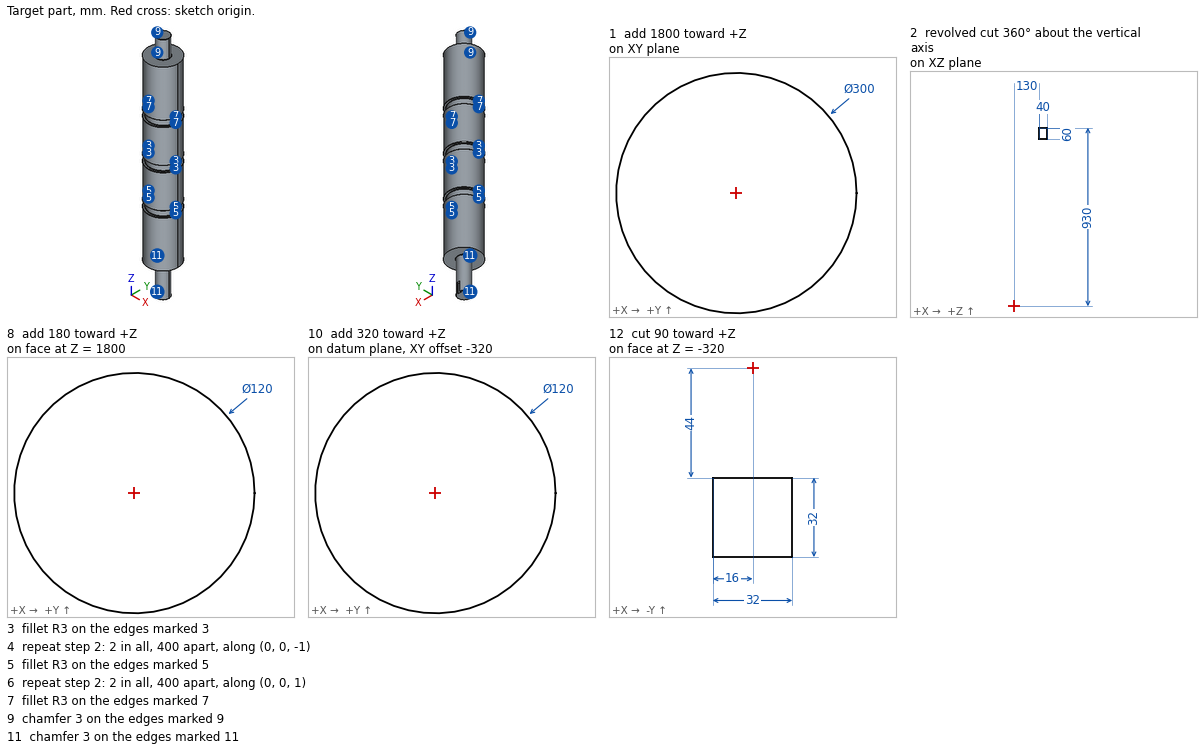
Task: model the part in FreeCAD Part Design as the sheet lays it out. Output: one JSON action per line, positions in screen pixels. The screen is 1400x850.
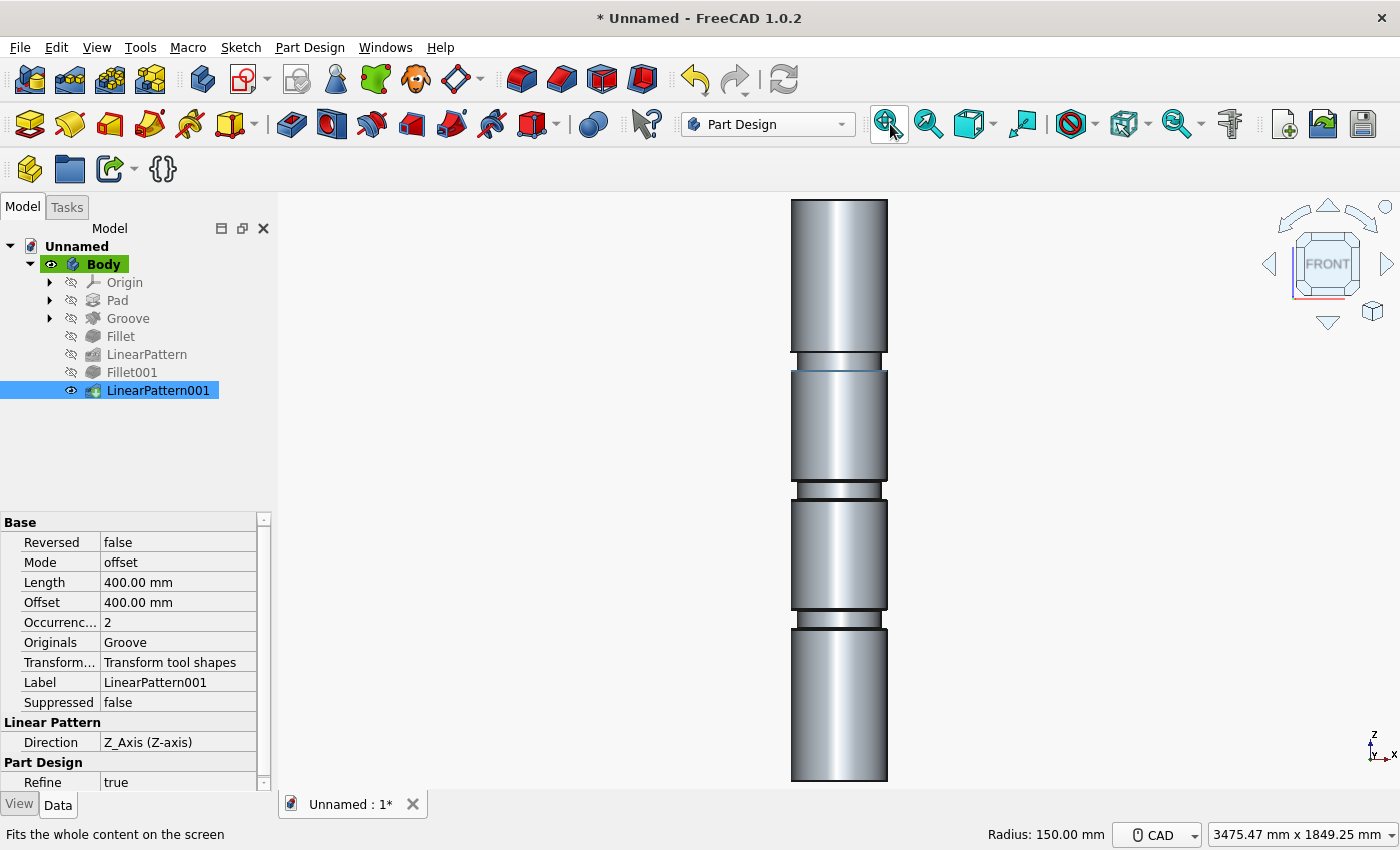
{"action": "left_click", "coordinate": [791, 351], "text": "ctrl"}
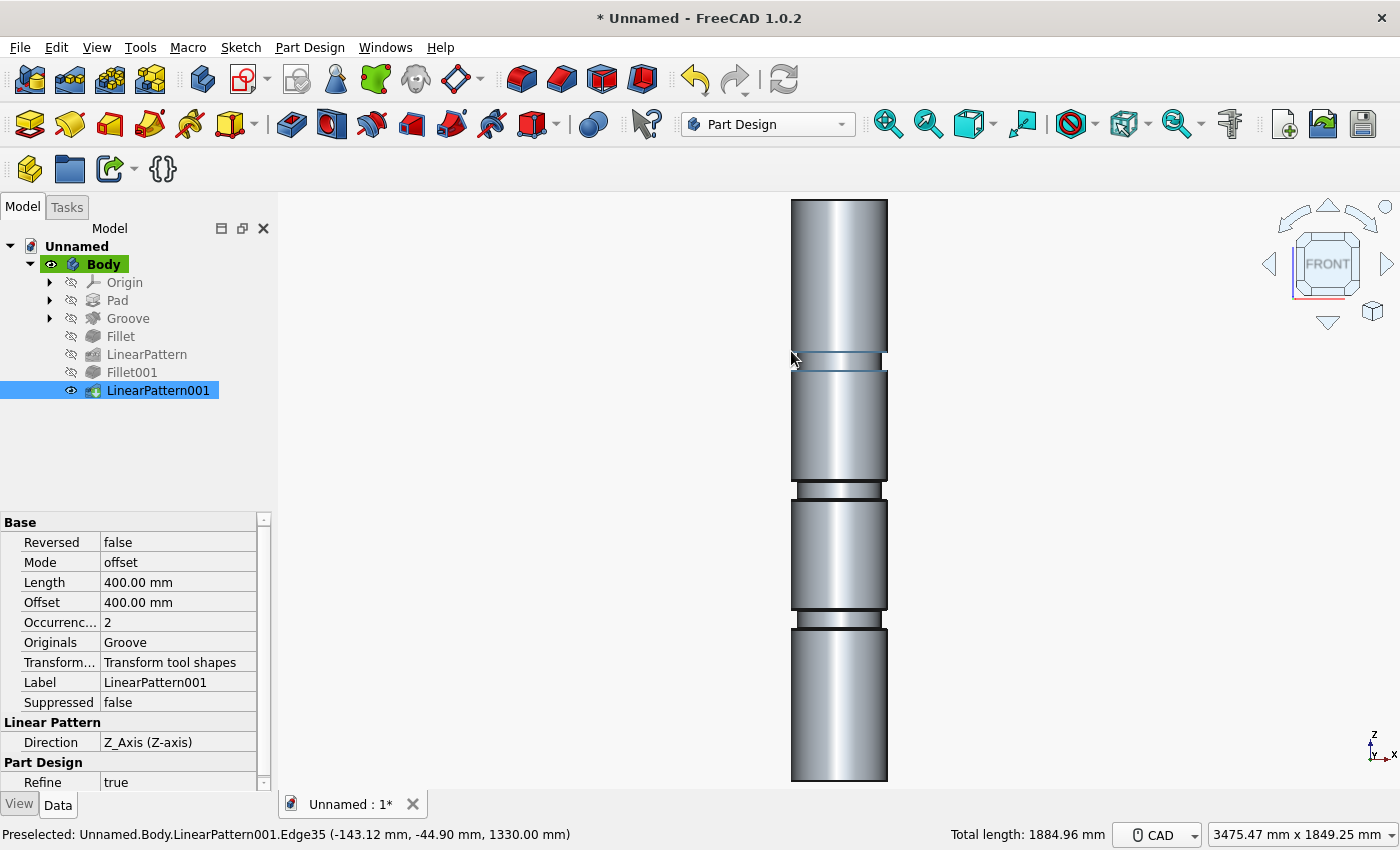
{"action": "key", "text": "3"}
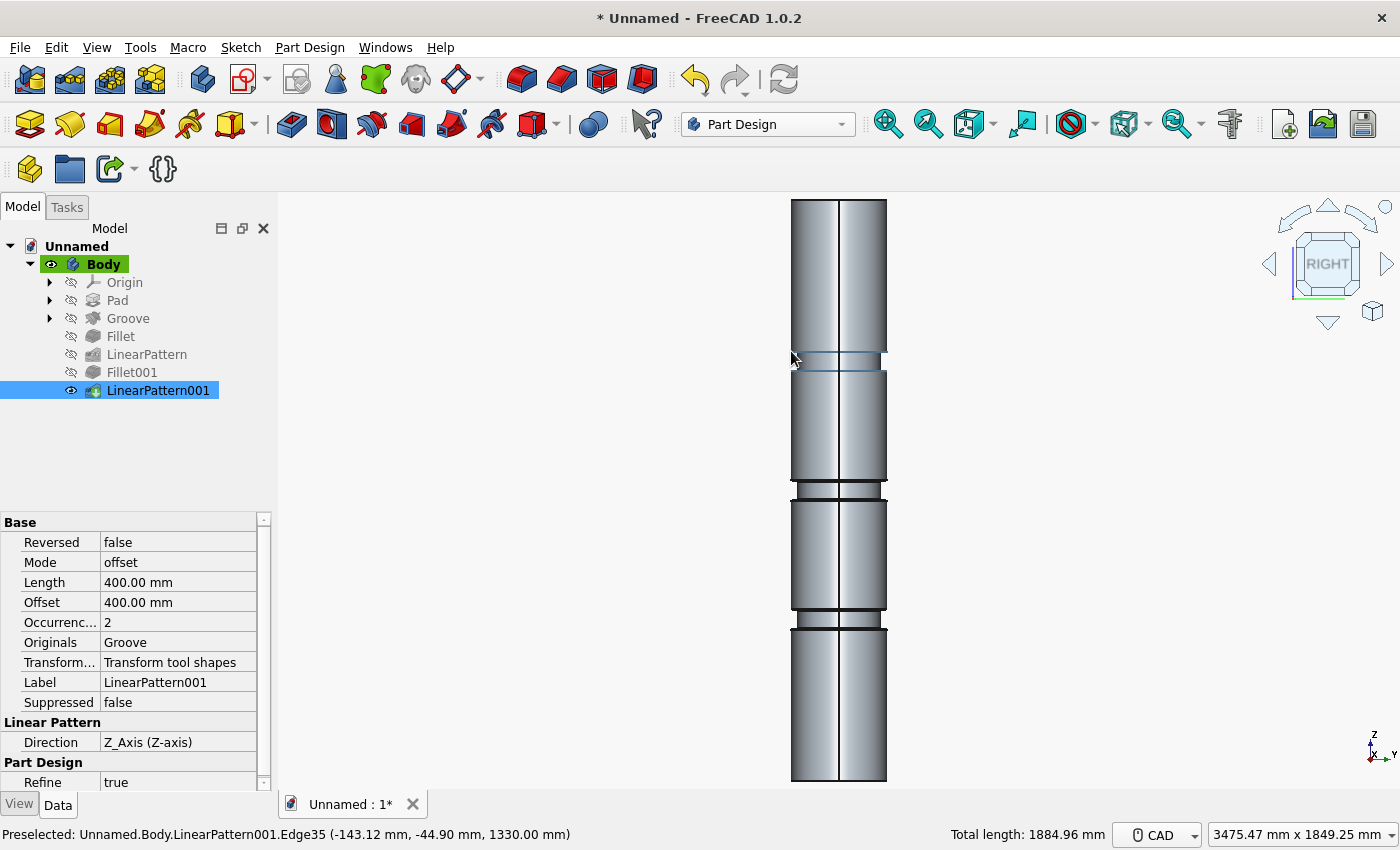
{"action": "key", "text": "5"}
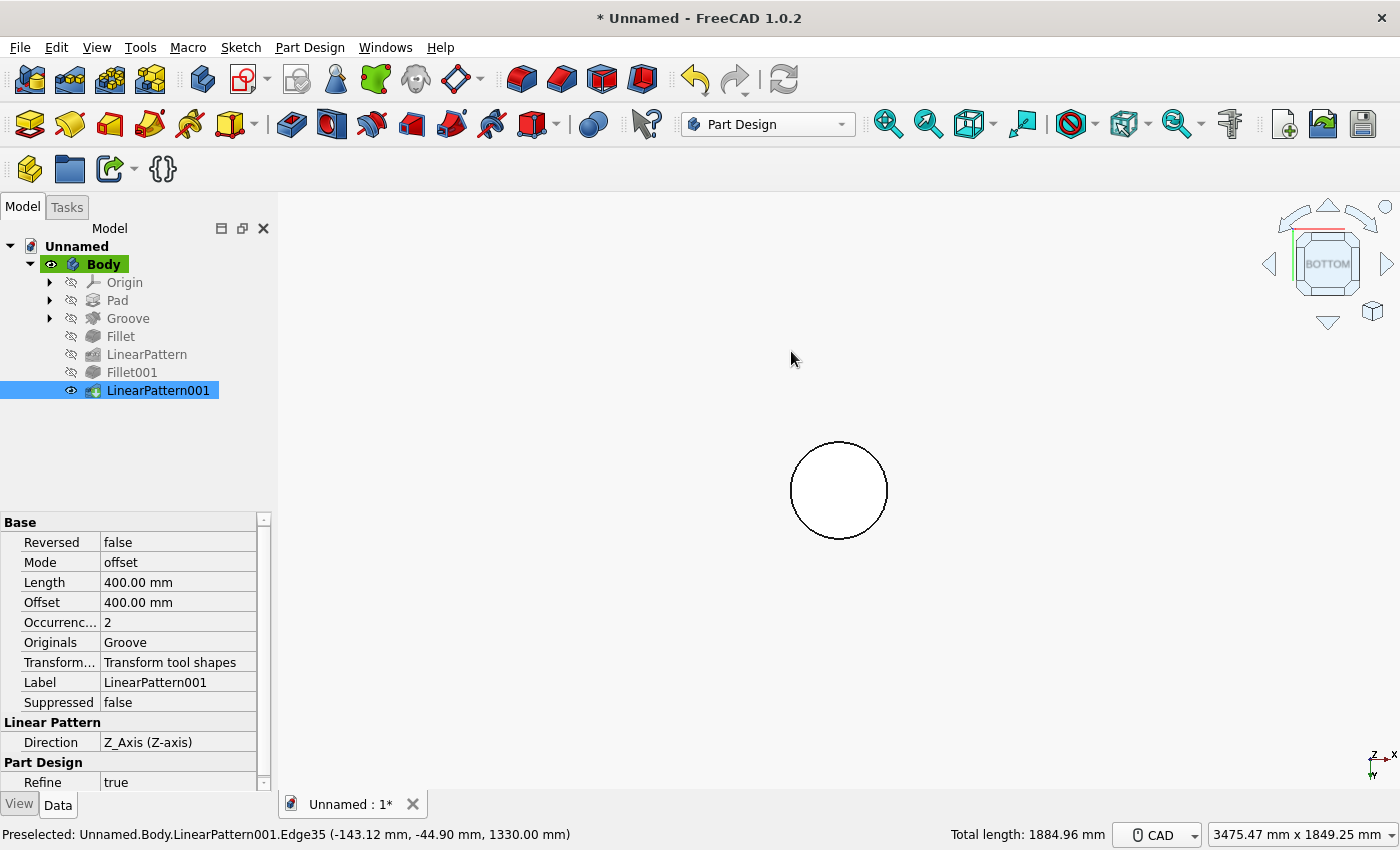
{"action": "left_click", "coordinate": [890, 124]}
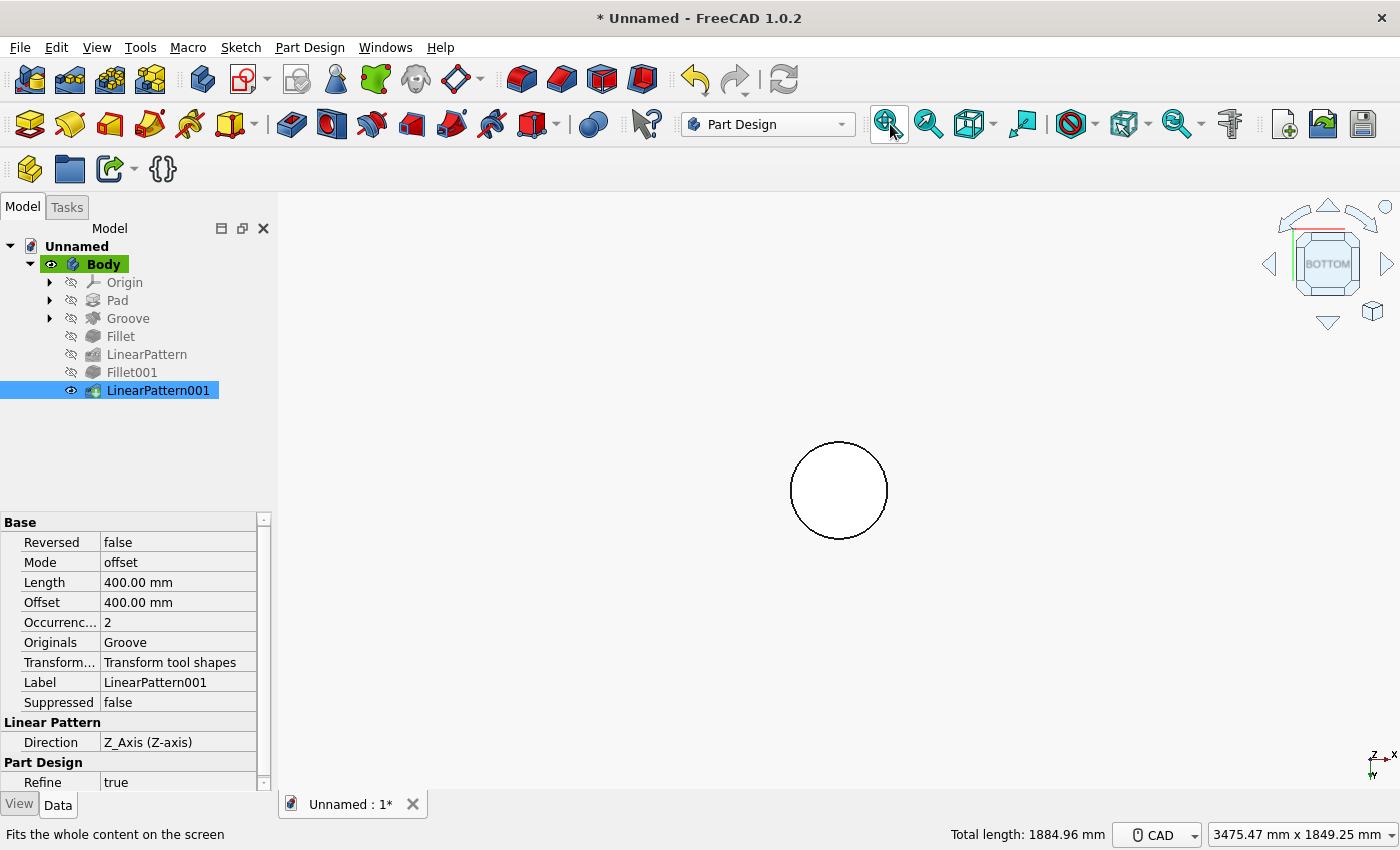
{"action": "key", "text": "4"}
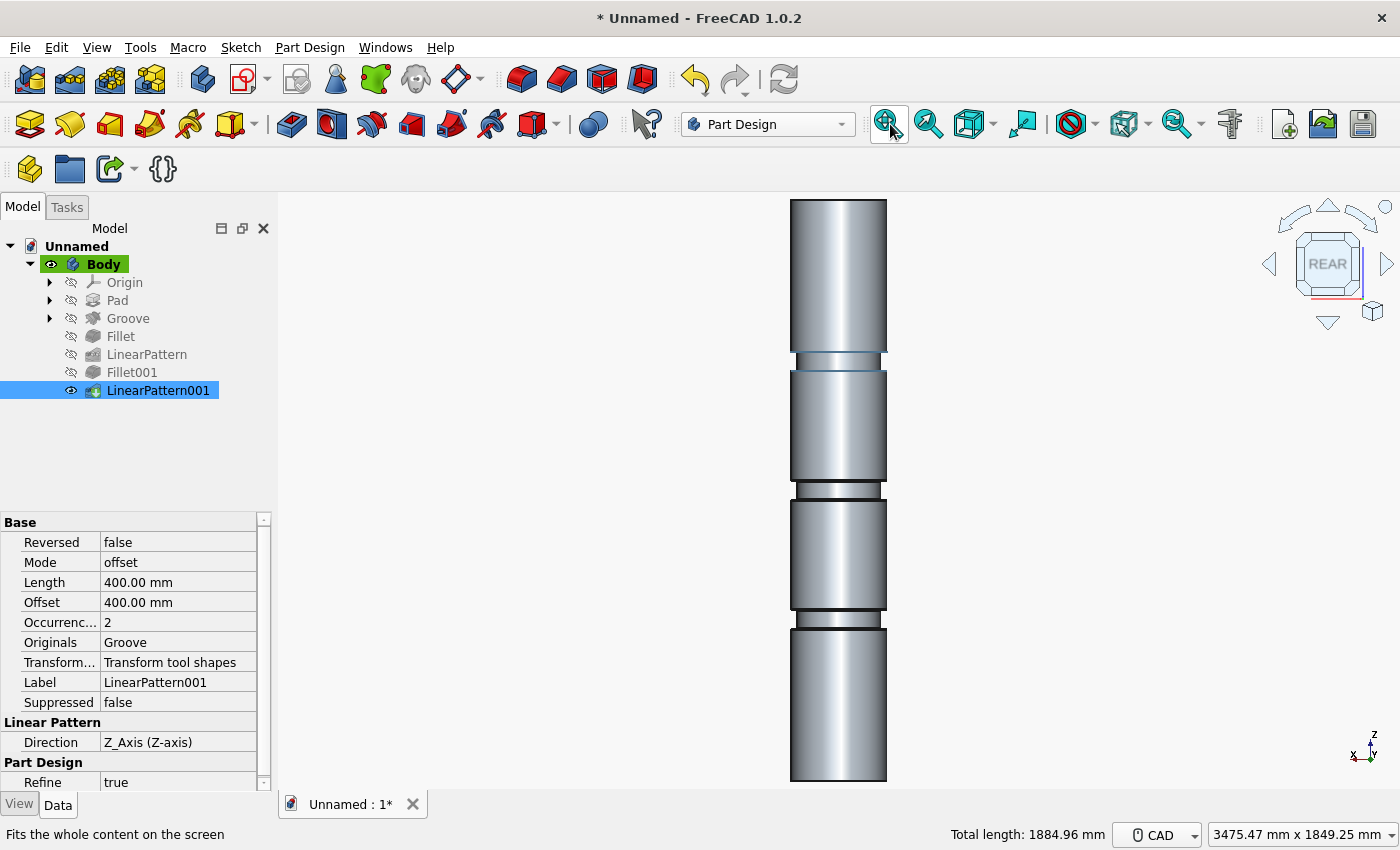
{"action": "key", "text": "6"}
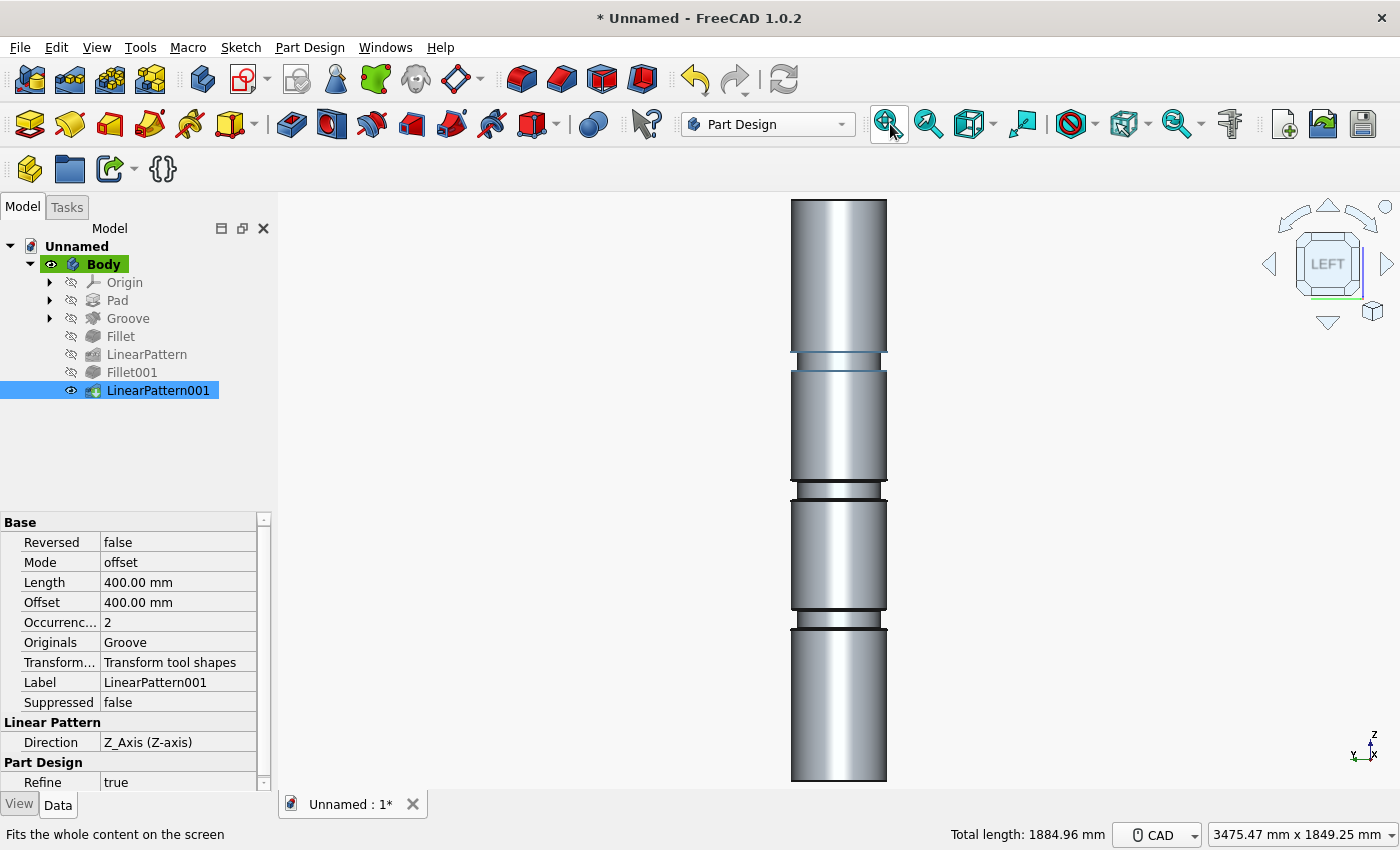
{"action": "key", "text": "v 3"}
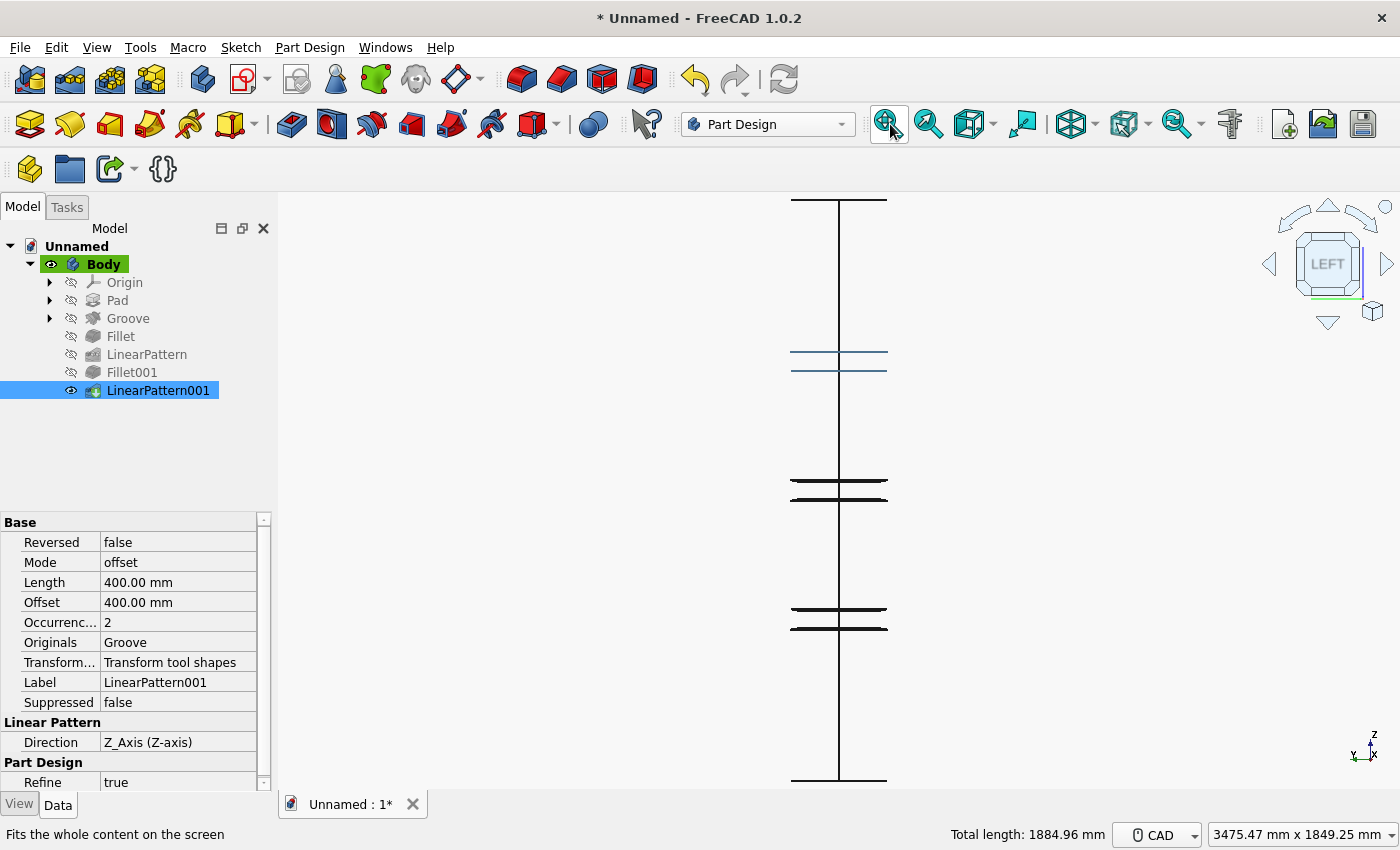
{"action": "key", "text": "0"}